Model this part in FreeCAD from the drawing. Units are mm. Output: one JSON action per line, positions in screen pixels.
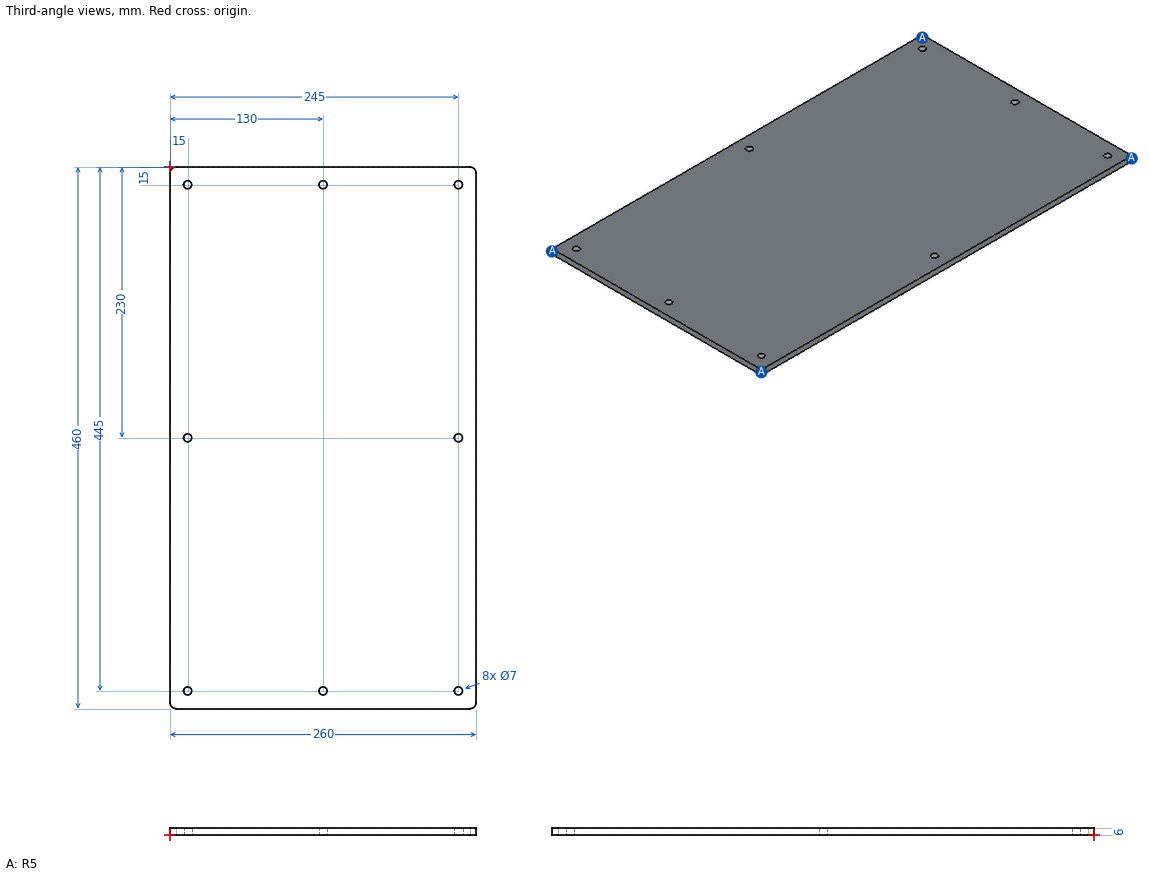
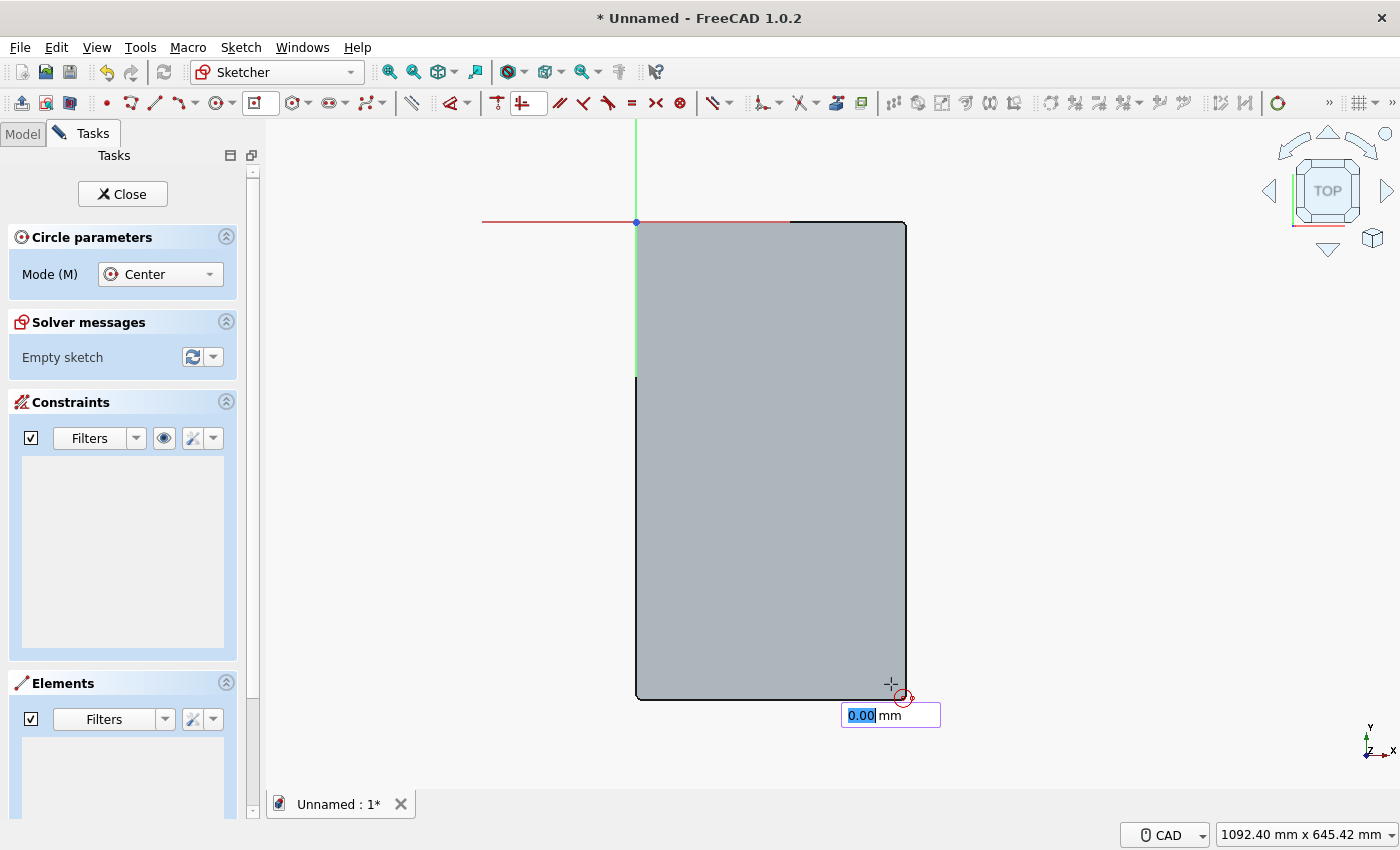
{"action": "scroll", "coordinate": [893, 682], "scroll_direction": "up", "scroll_amount": 8}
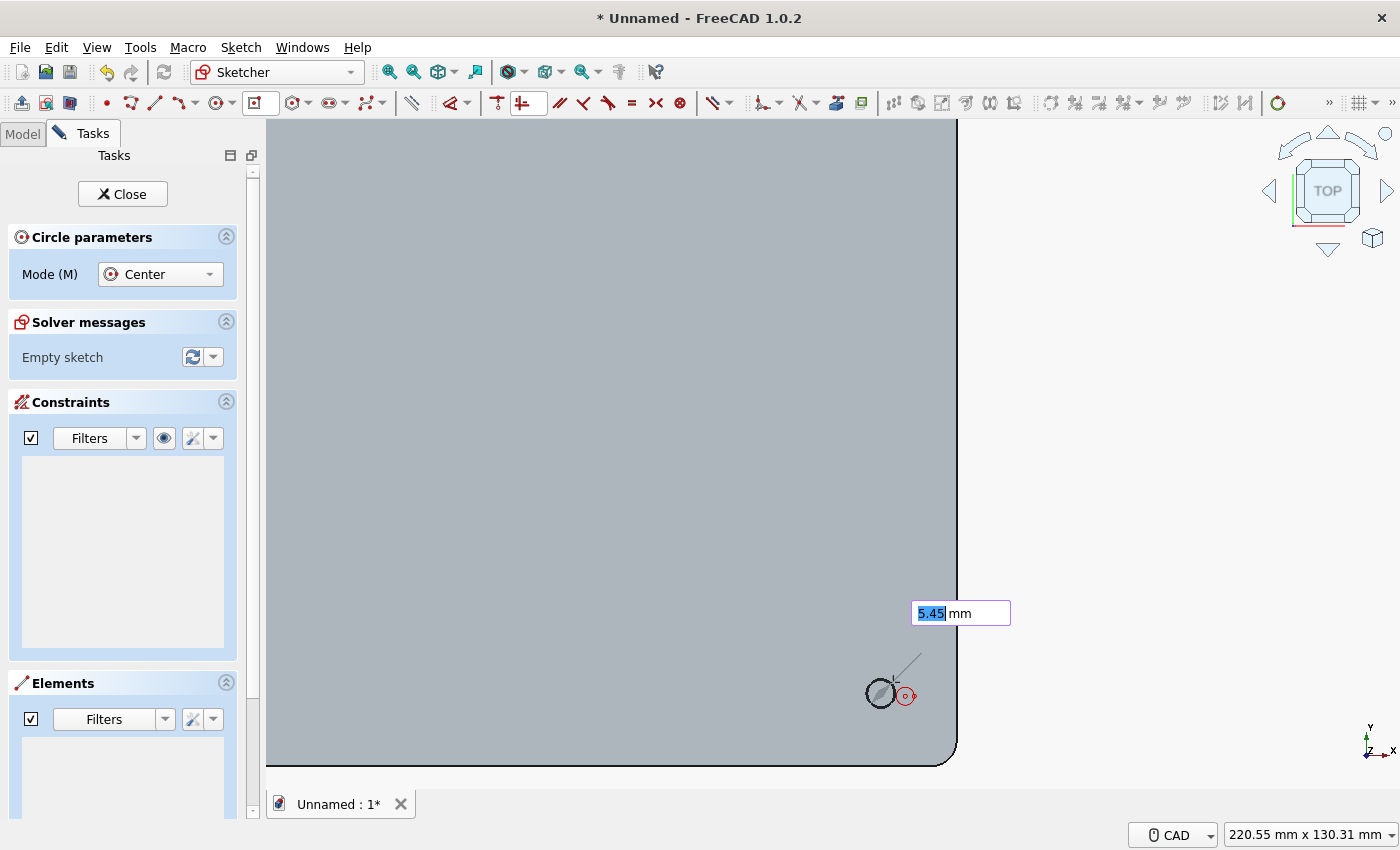
{"action": "left_click", "coordinate": [892, 677]}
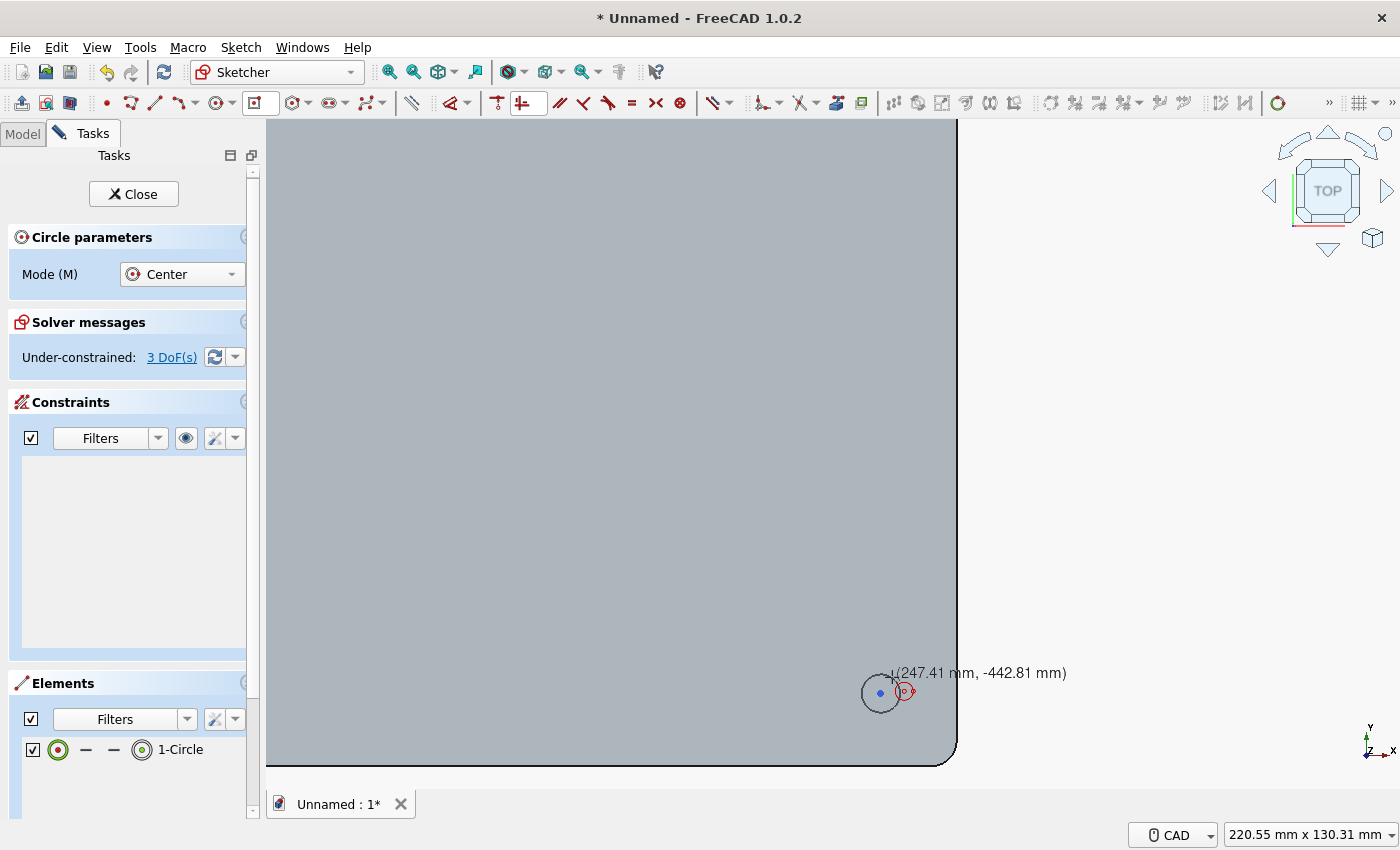
{"action": "scroll", "coordinate": [892, 682], "scroll_direction": "down", "scroll_amount": 8}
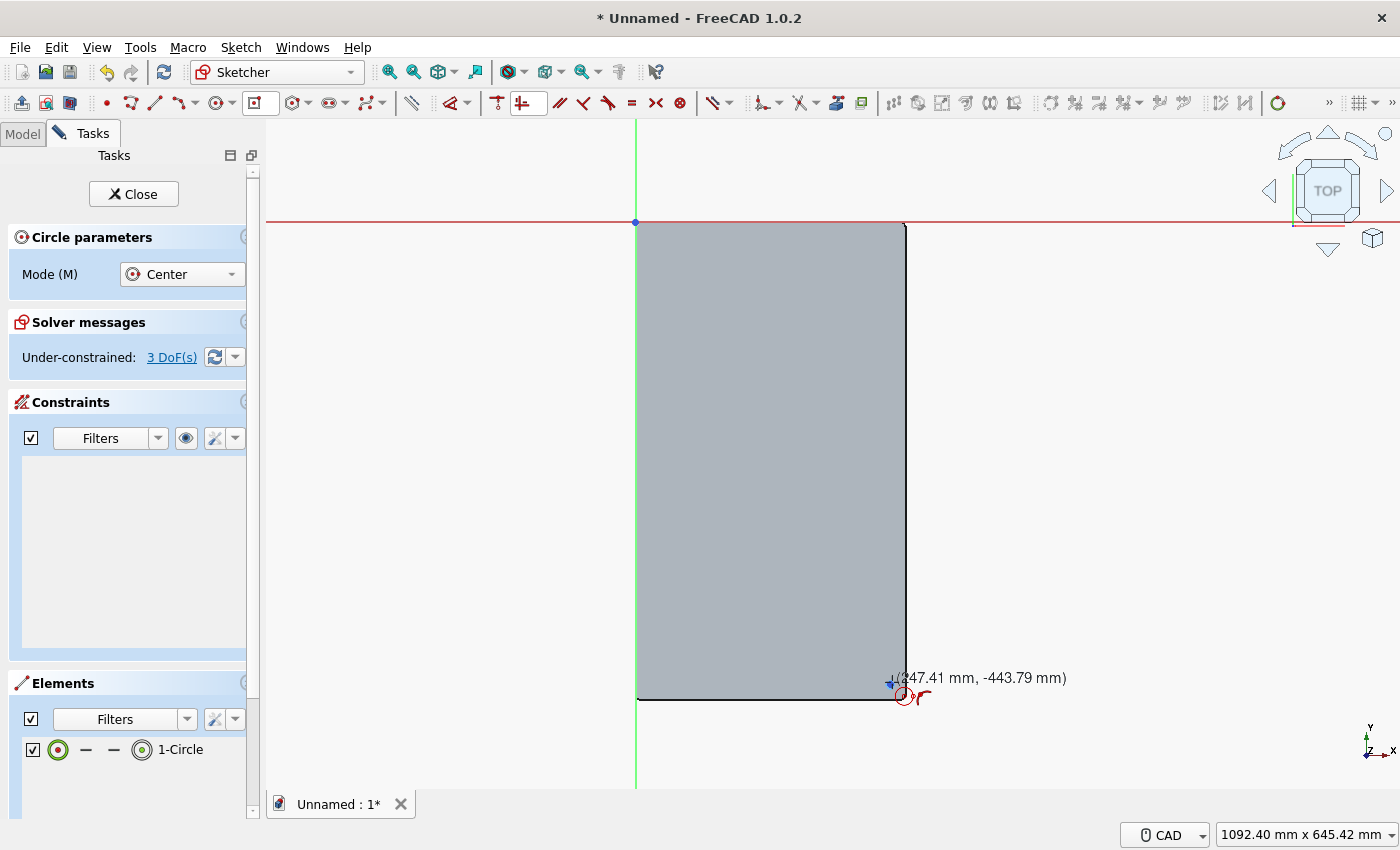
{"action": "scroll", "coordinate": [651, 684], "scroll_direction": "up", "scroll_amount": 10}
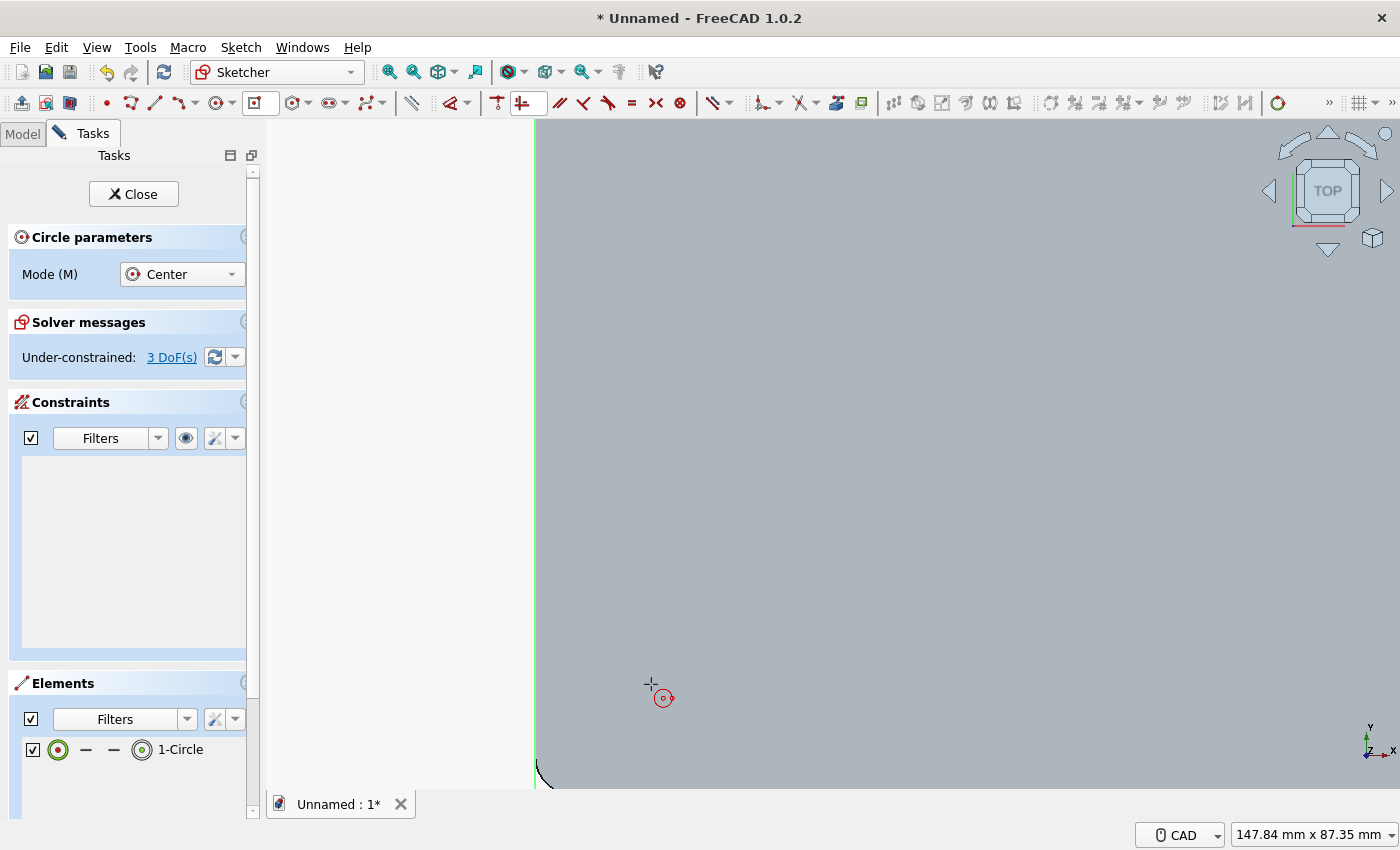
{"action": "scroll", "coordinate": [651, 684], "scroll_direction": "down", "scroll_amount": 10}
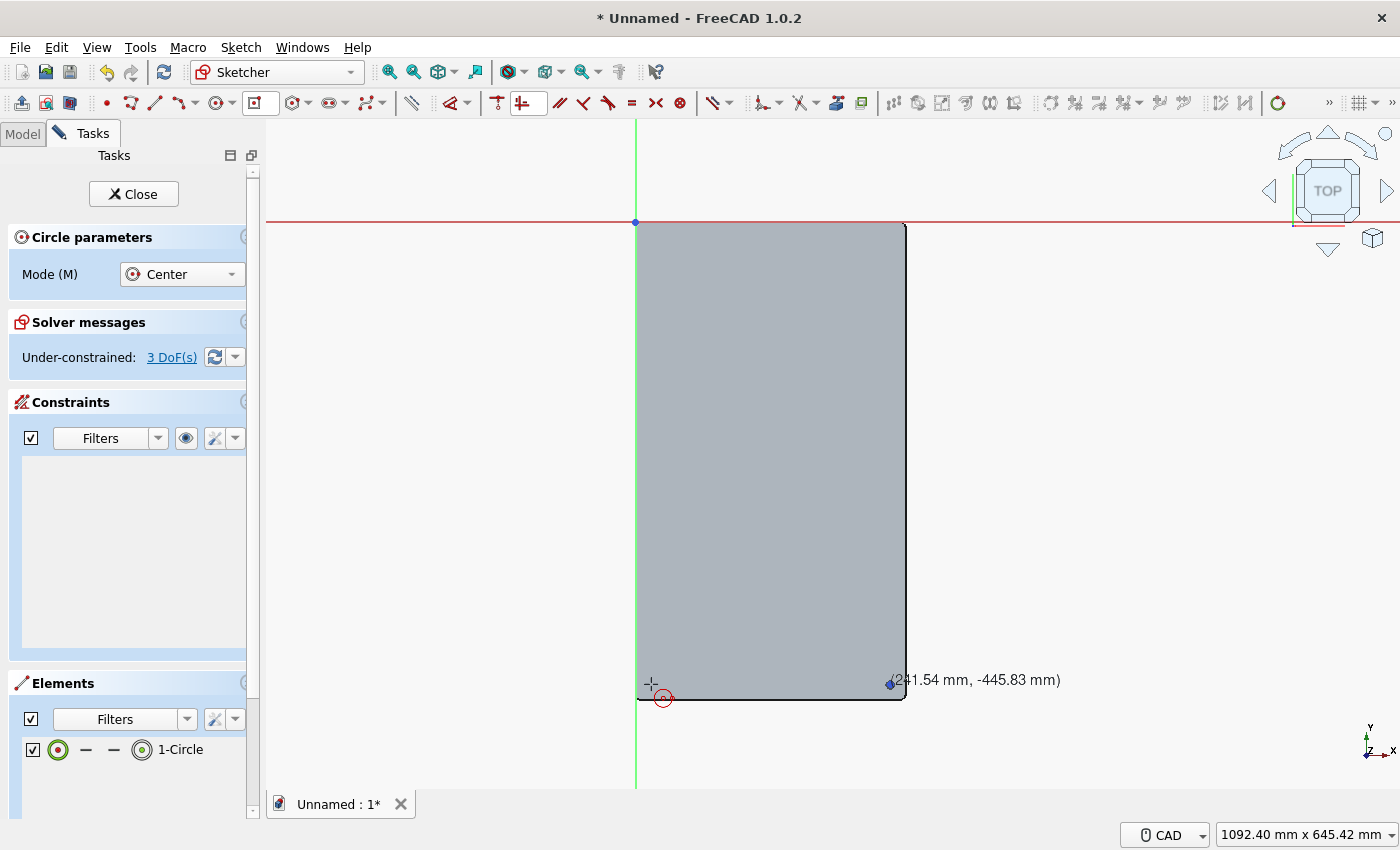
{"action": "left_click", "coordinate": [651, 684]}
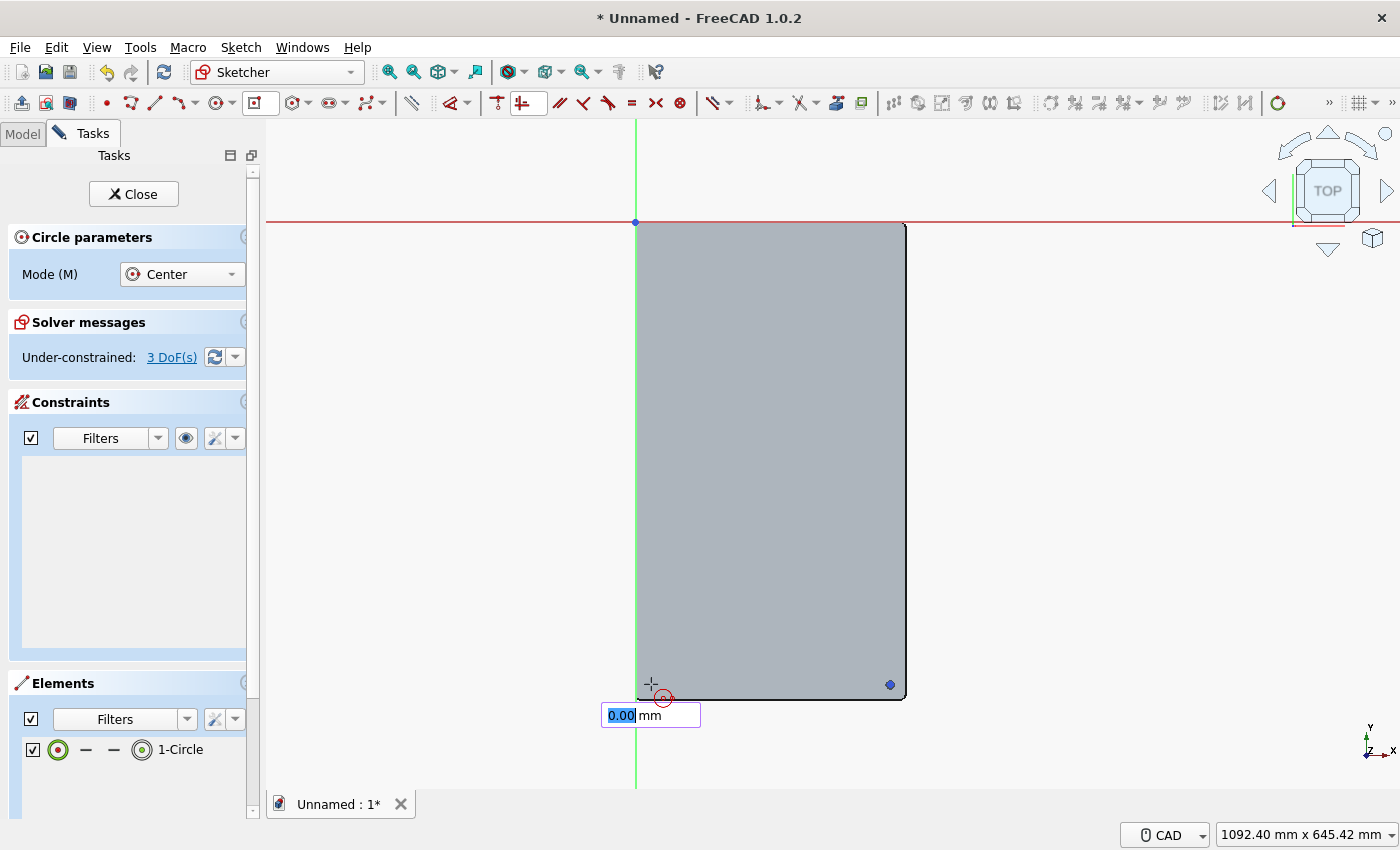
{"action": "scroll", "coordinate": [654, 682], "scroll_direction": "up", "scroll_amount": 8}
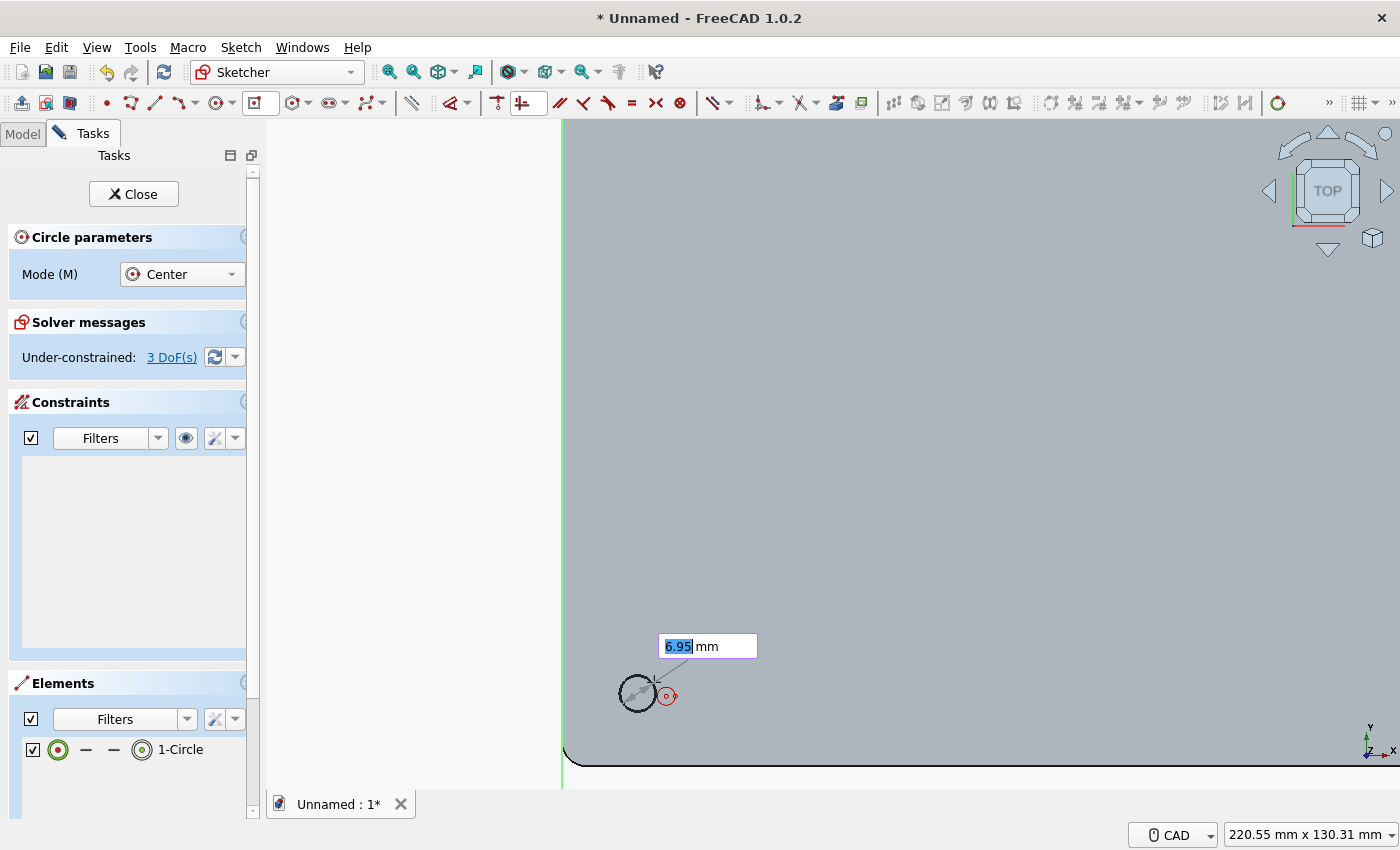
{"action": "left_click", "coordinate": [651, 677]}